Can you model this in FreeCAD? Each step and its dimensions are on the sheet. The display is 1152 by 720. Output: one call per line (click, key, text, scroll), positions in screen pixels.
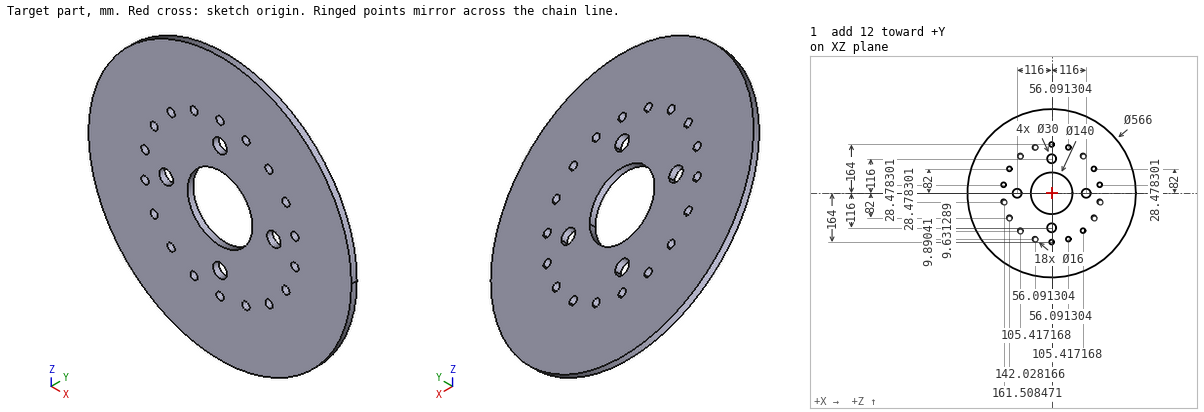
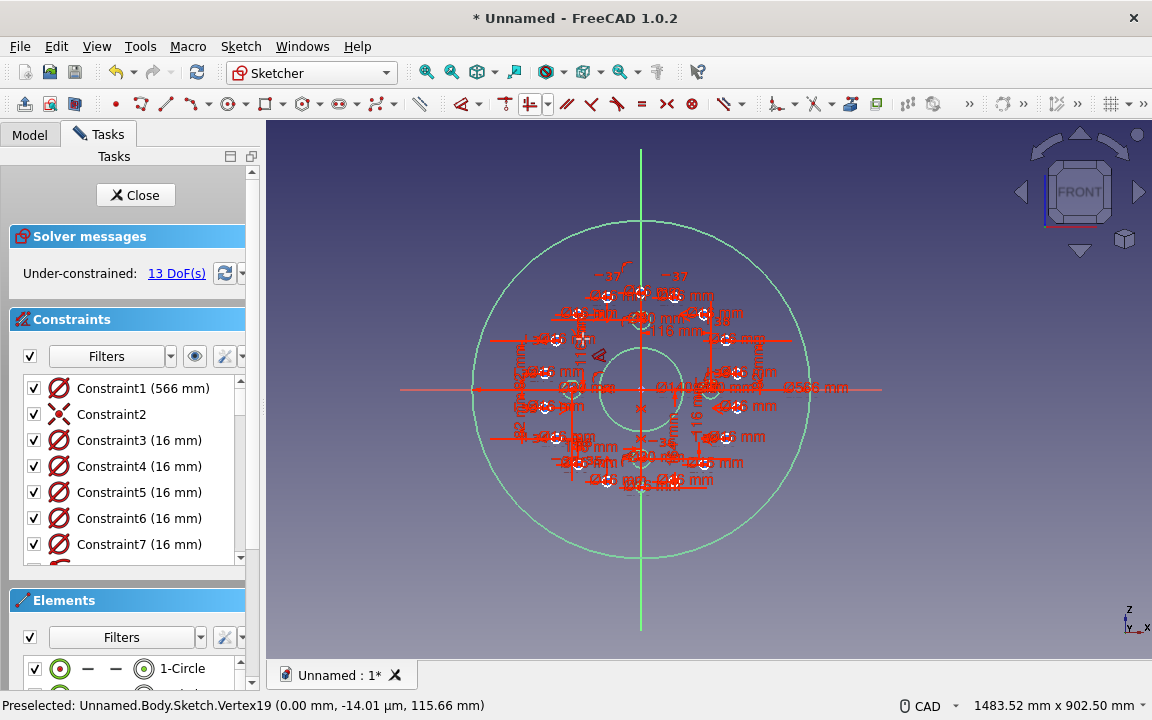
click(641, 293)
click(723, 308)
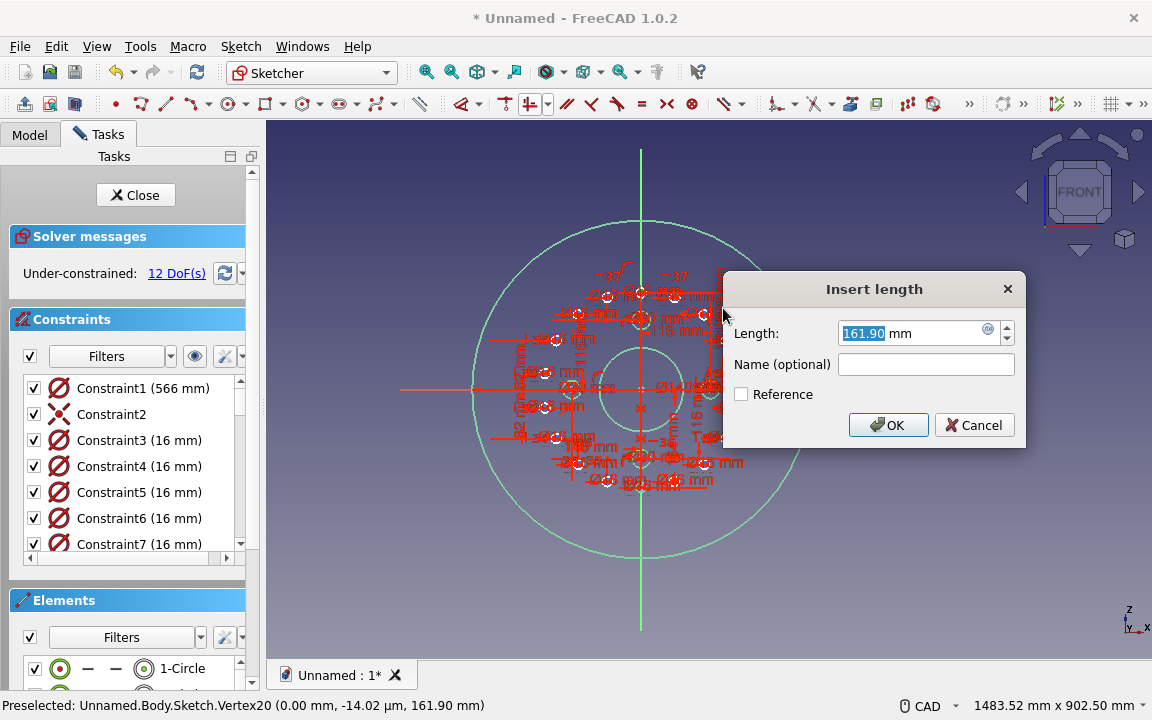
text(164)
key(Return)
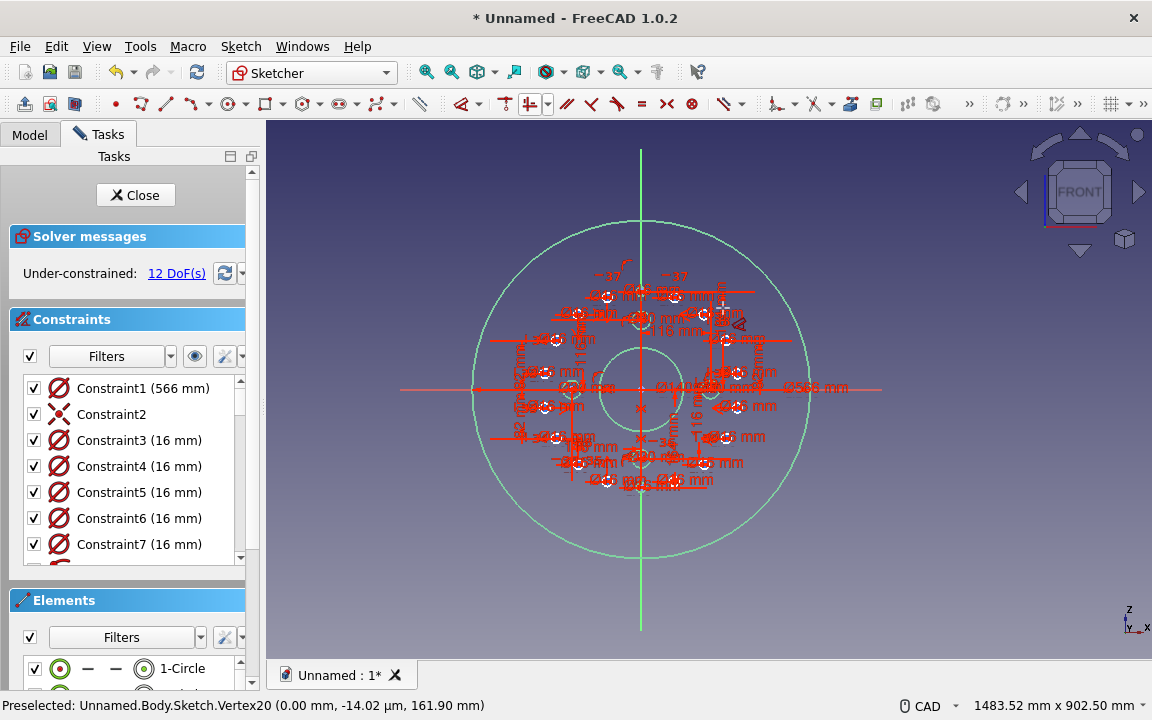
scroll(607, 482, up, 10)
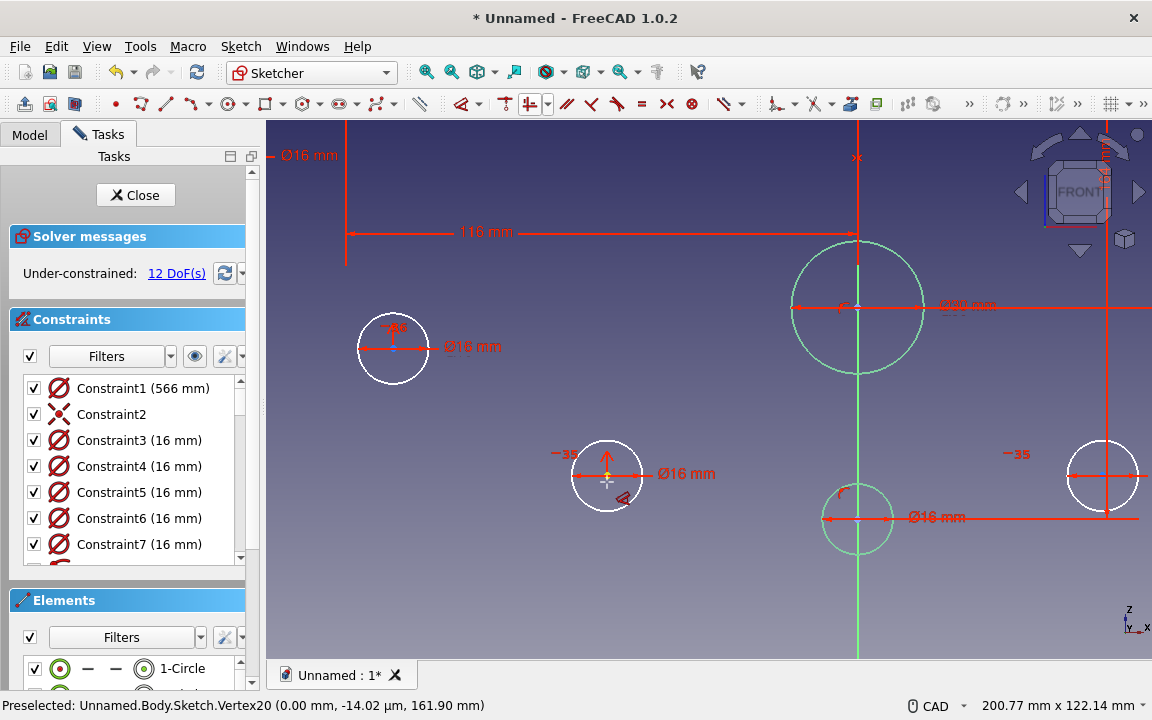
click(607, 476)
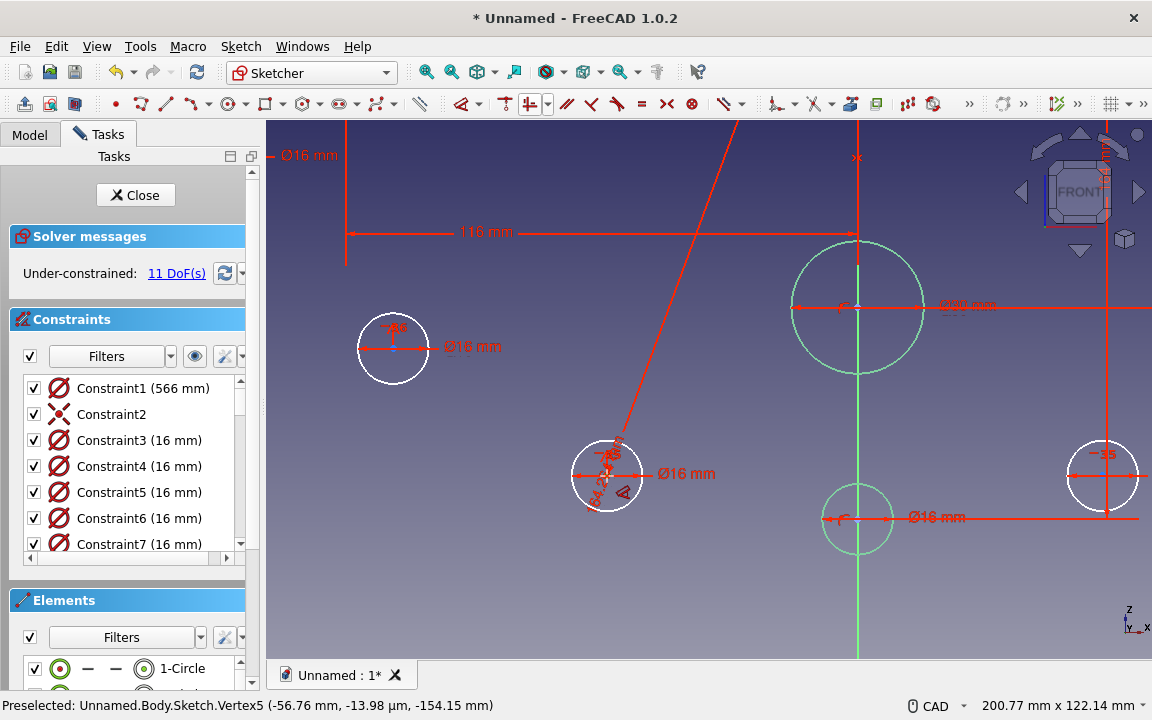
click(858, 519)
click(573, 513)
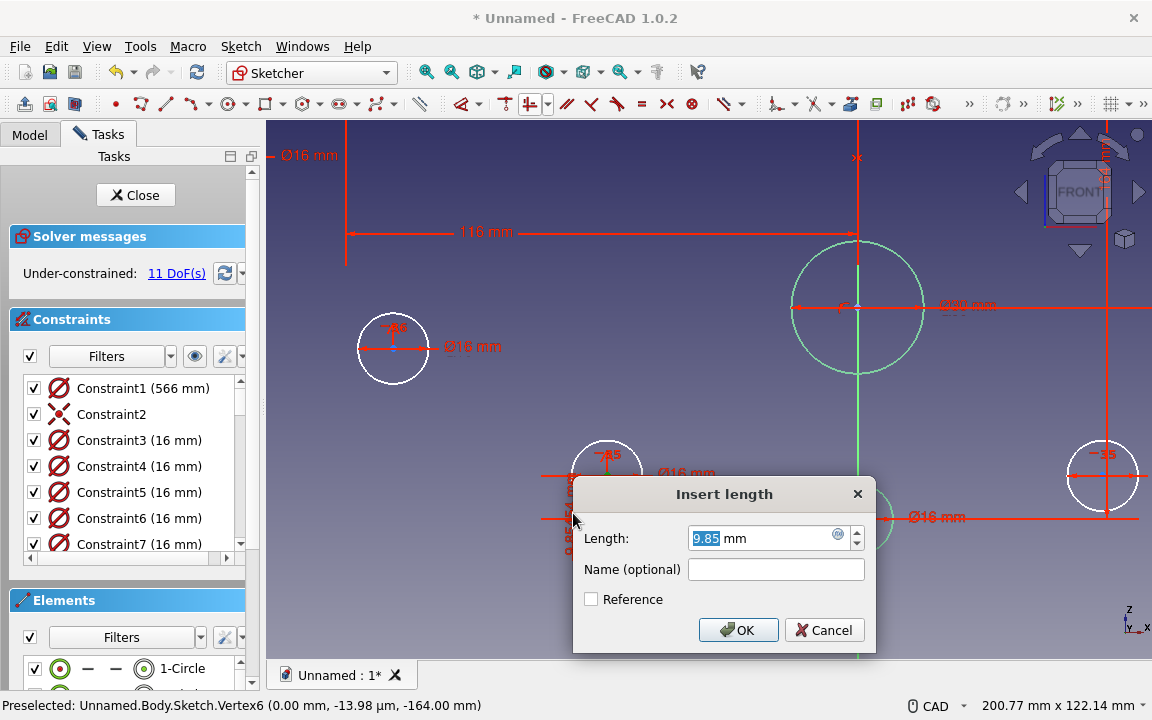
text(9.89041)
key(Return)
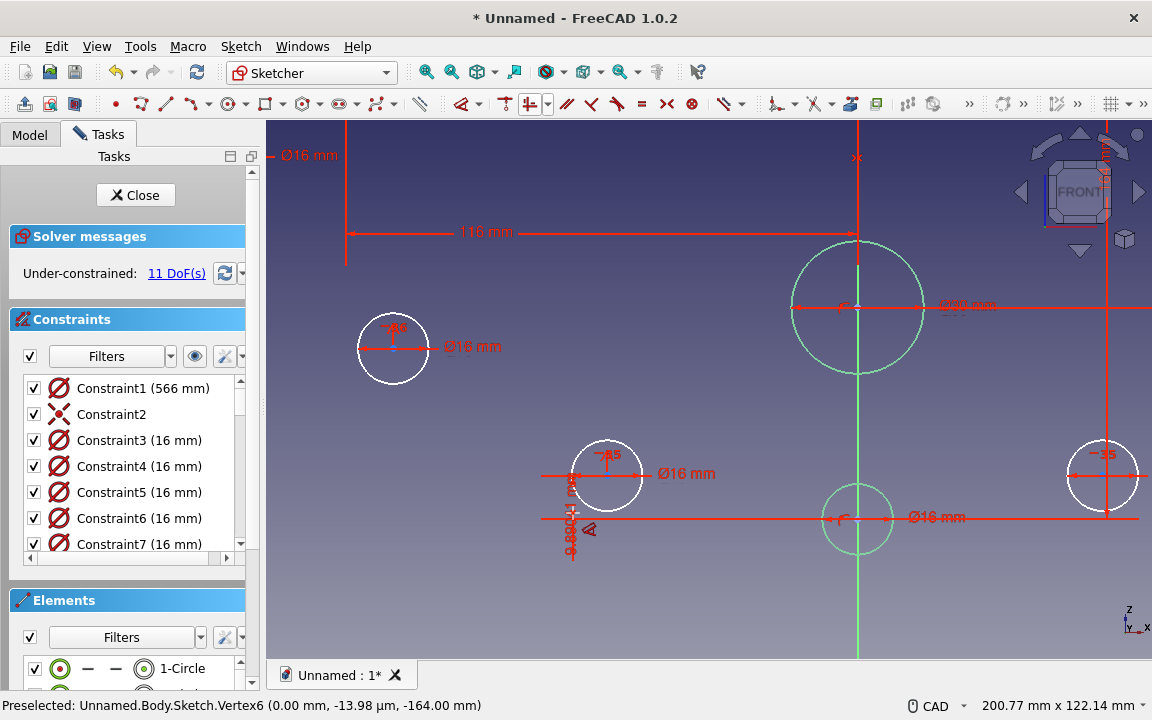
scroll(607, 482, down, 10)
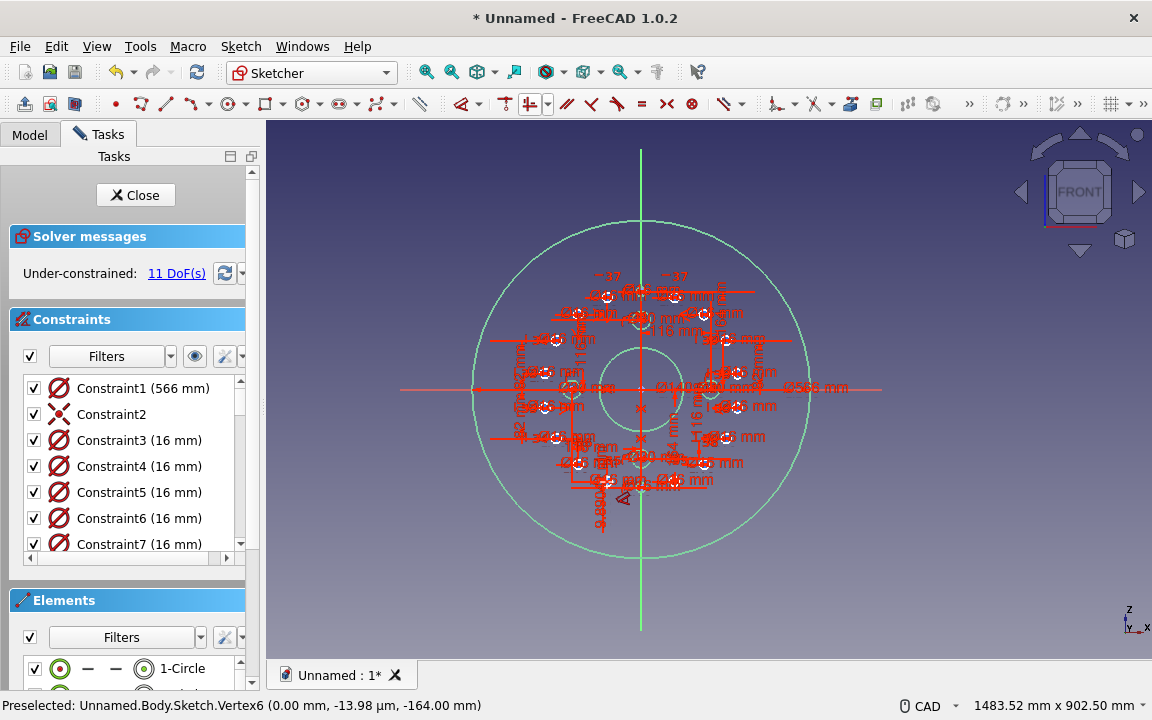
scroll(545, 408, up, 5)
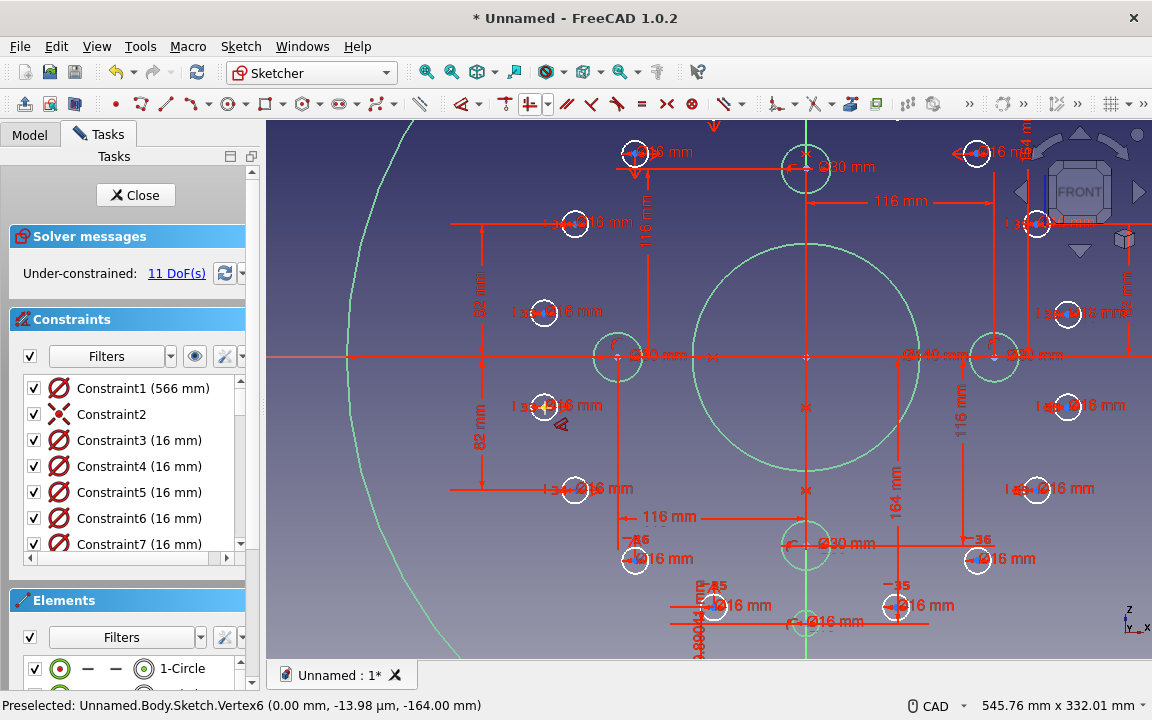
click(544, 407)
click(510, 382)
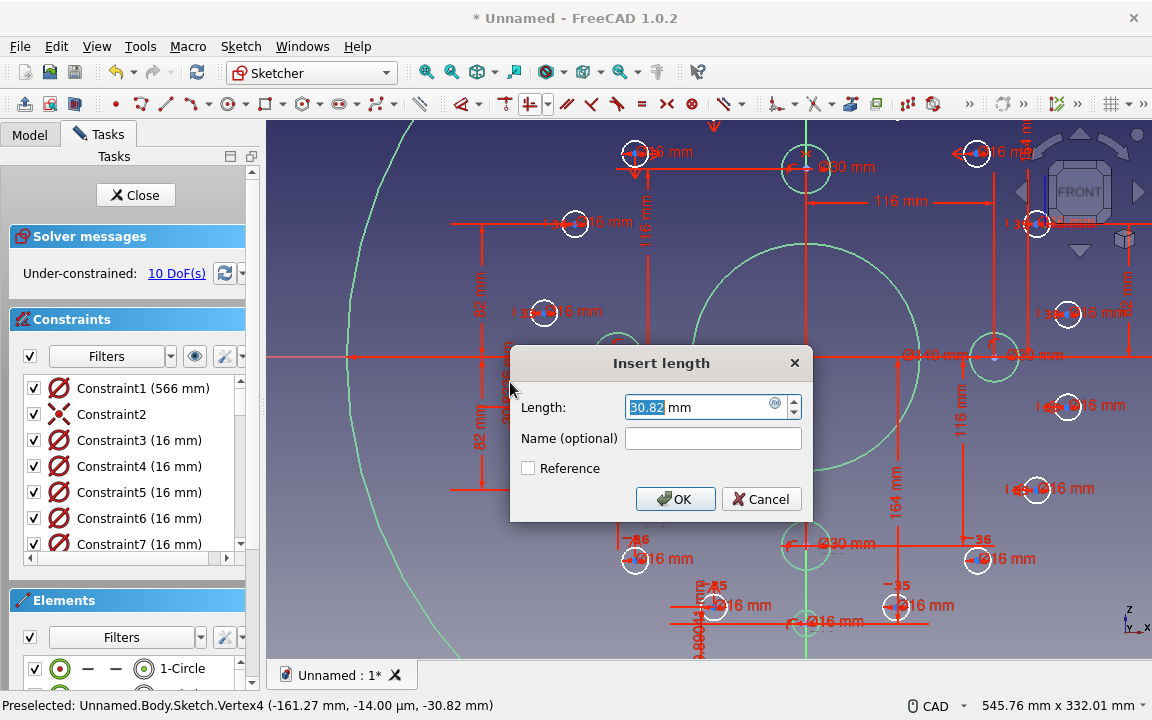
text(28.478301)
key(Return)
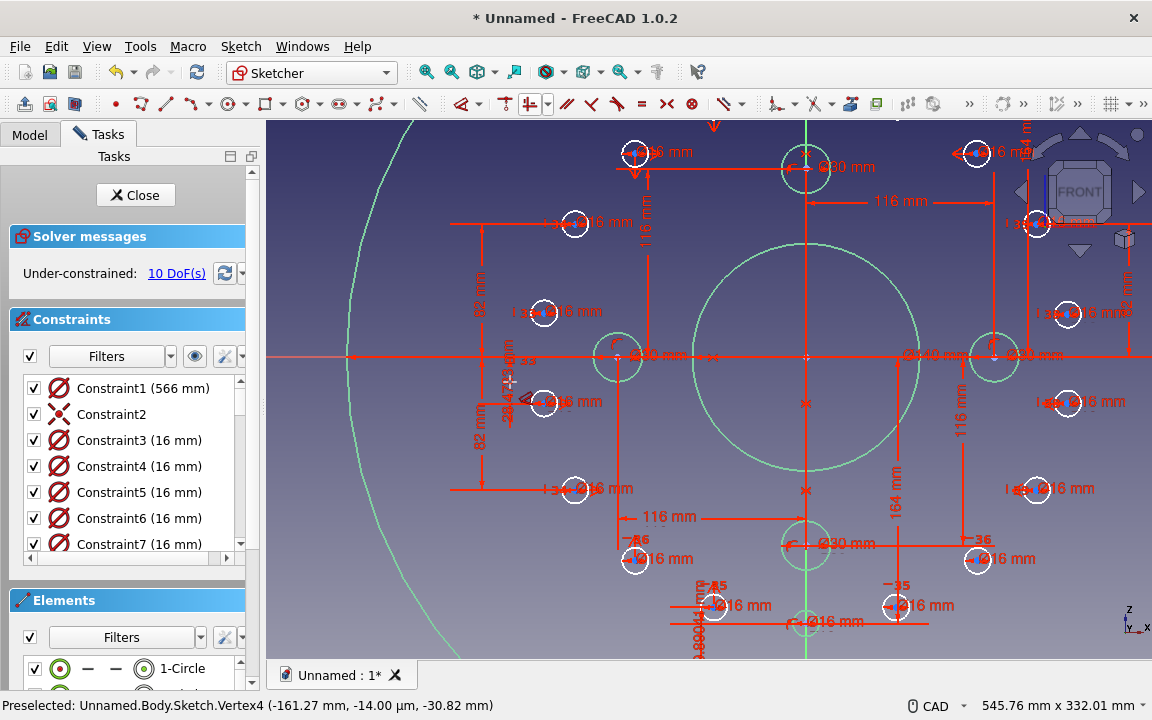
click(714, 607)
click(760, 323)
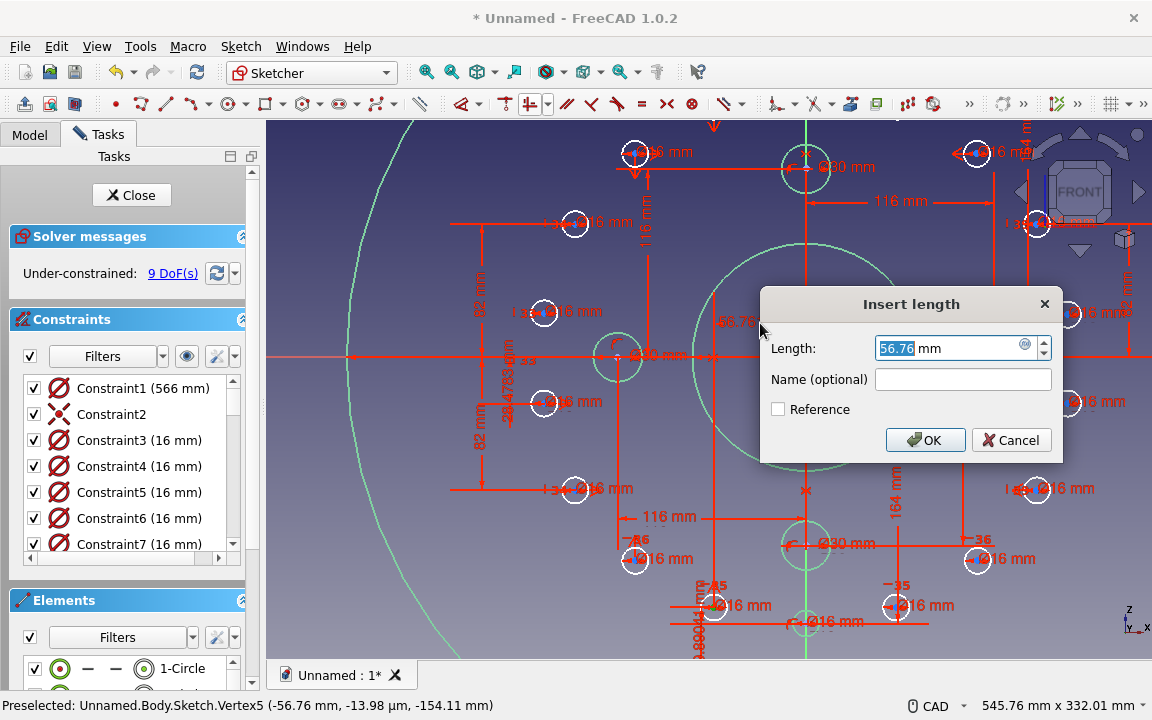
text(56.091304)
key(Return)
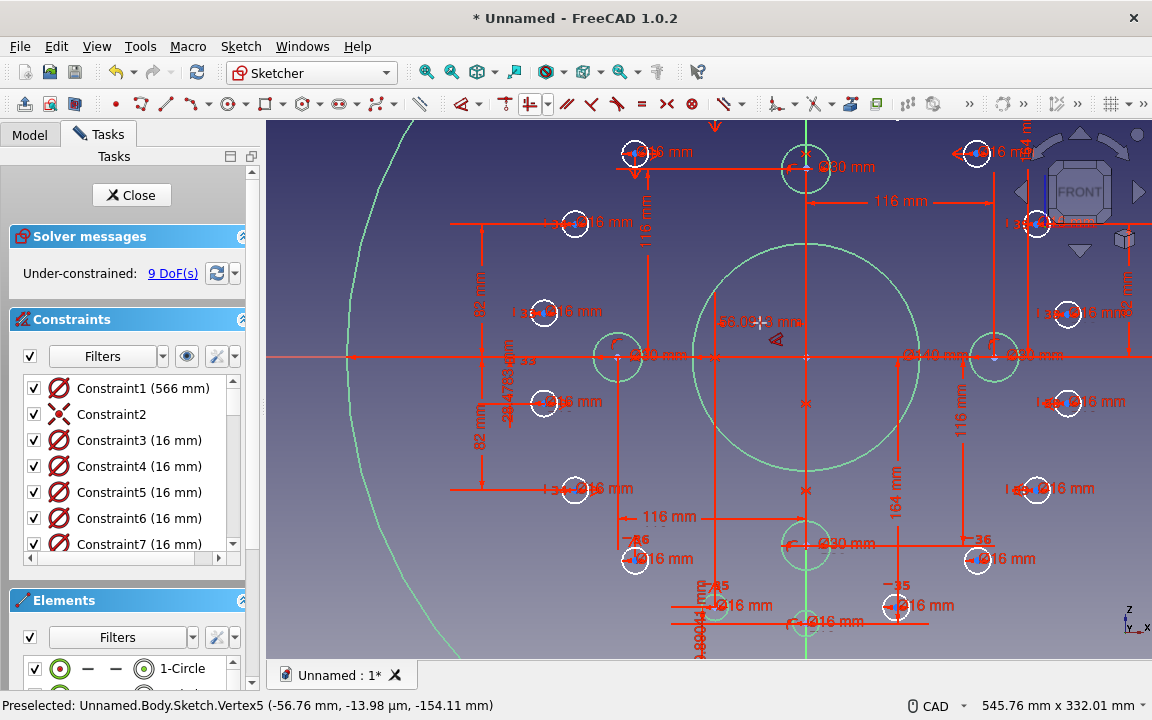
click(544, 313)
click(510, 335)